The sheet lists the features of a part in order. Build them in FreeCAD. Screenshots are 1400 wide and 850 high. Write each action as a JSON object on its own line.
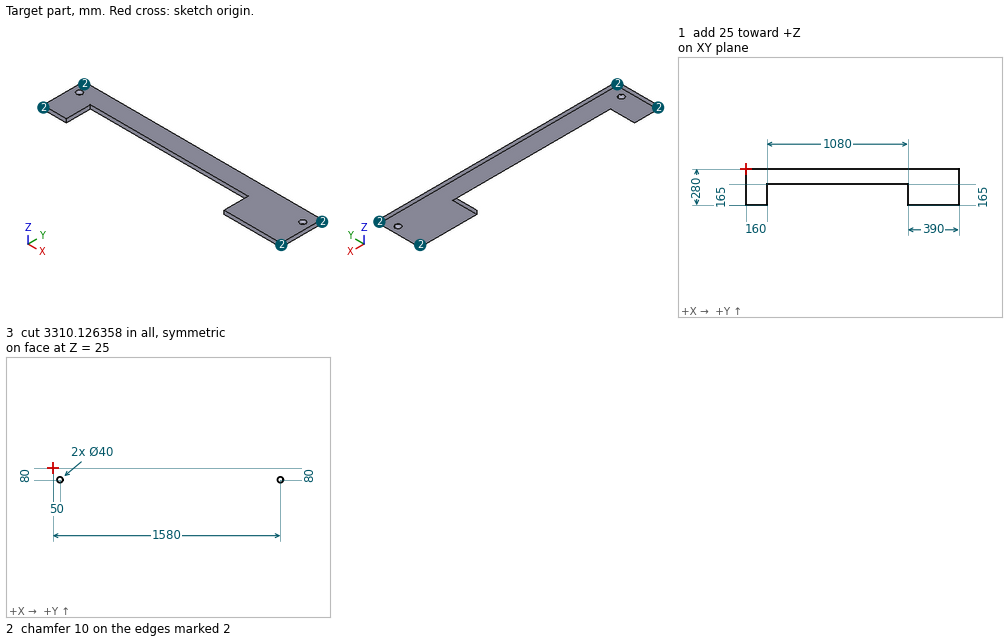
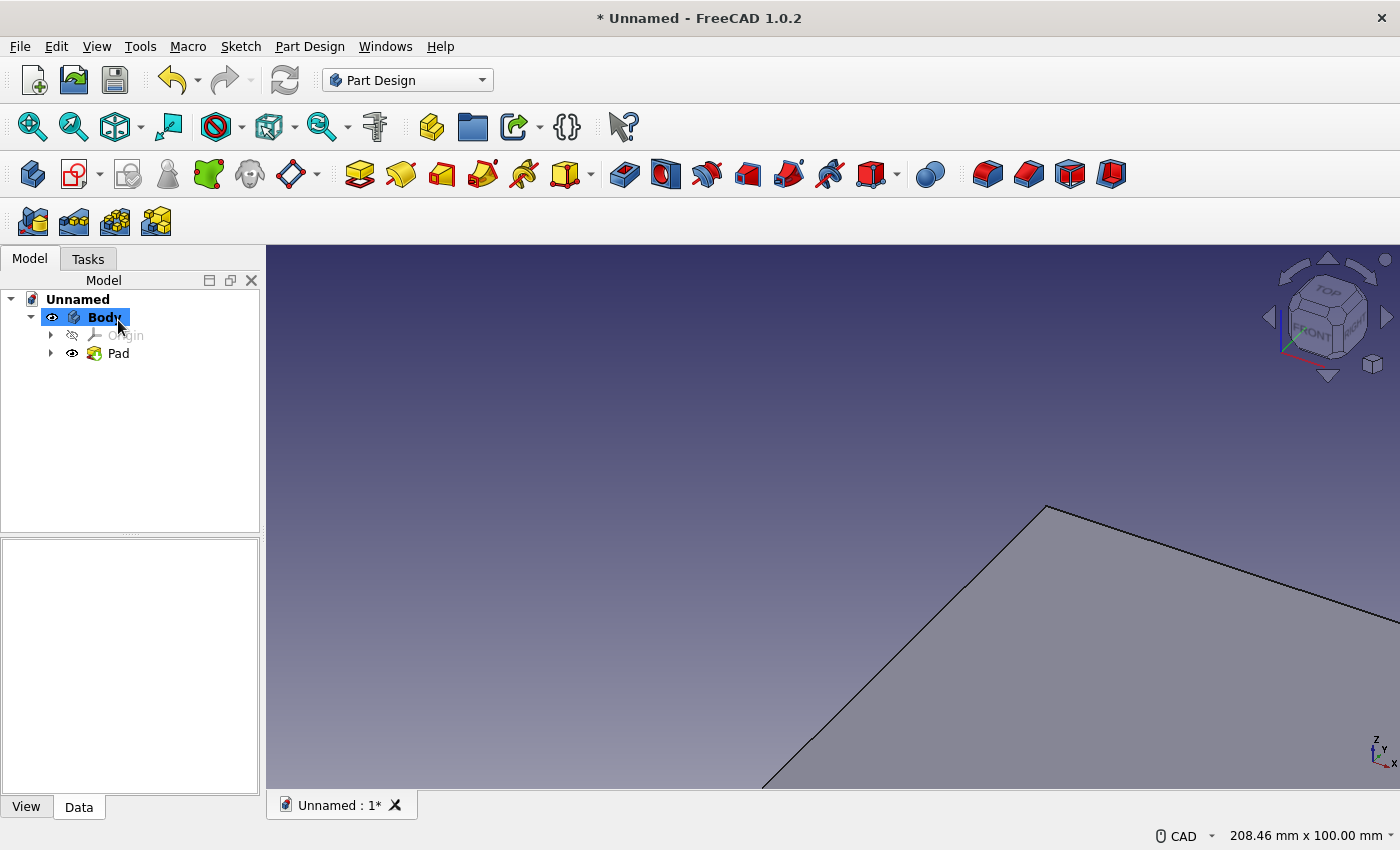
{"action": "key", "text": "v f"}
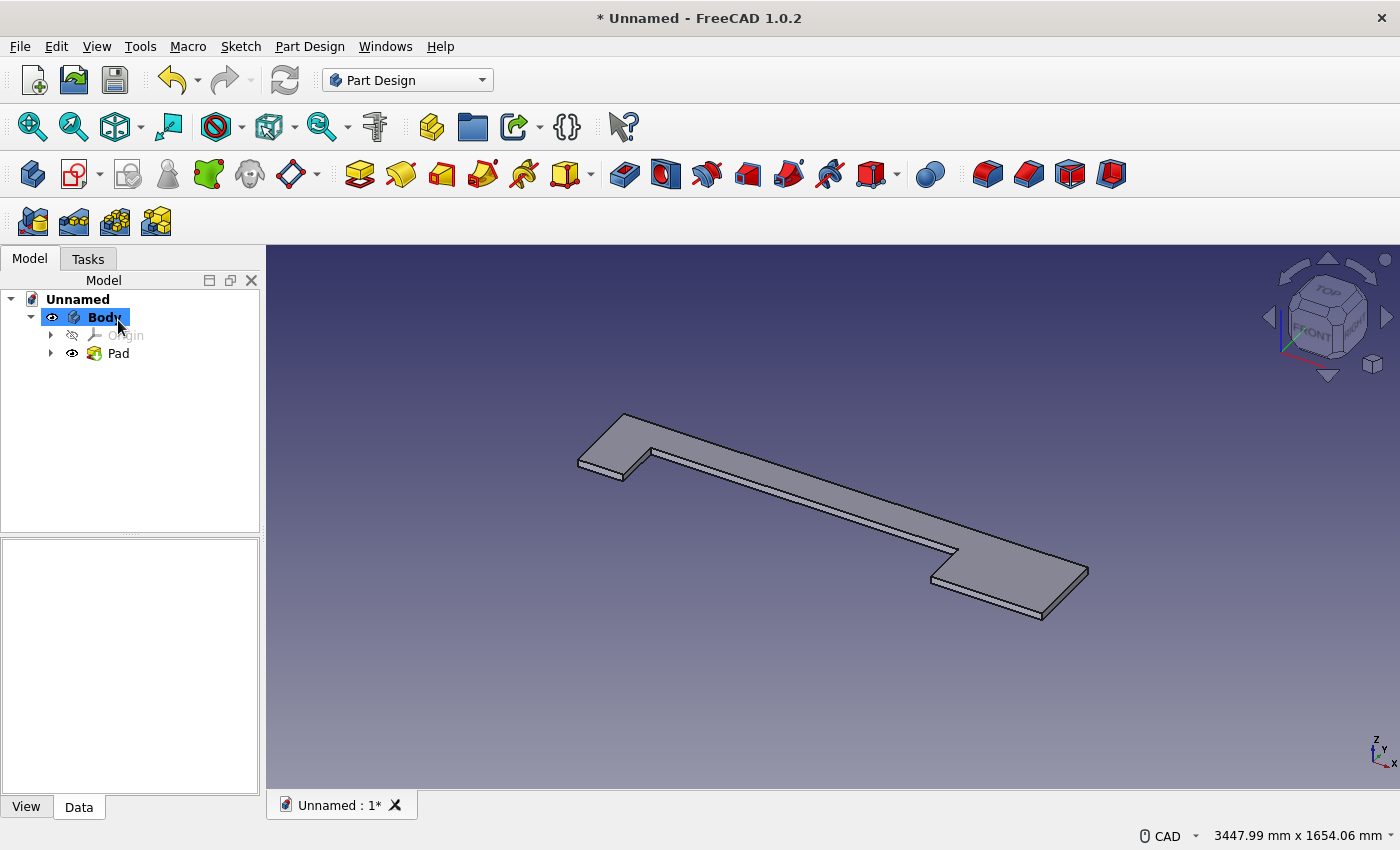
{"action": "scroll", "coordinate": [578, 462], "scroll_direction": "up", "scroll_amount": 8}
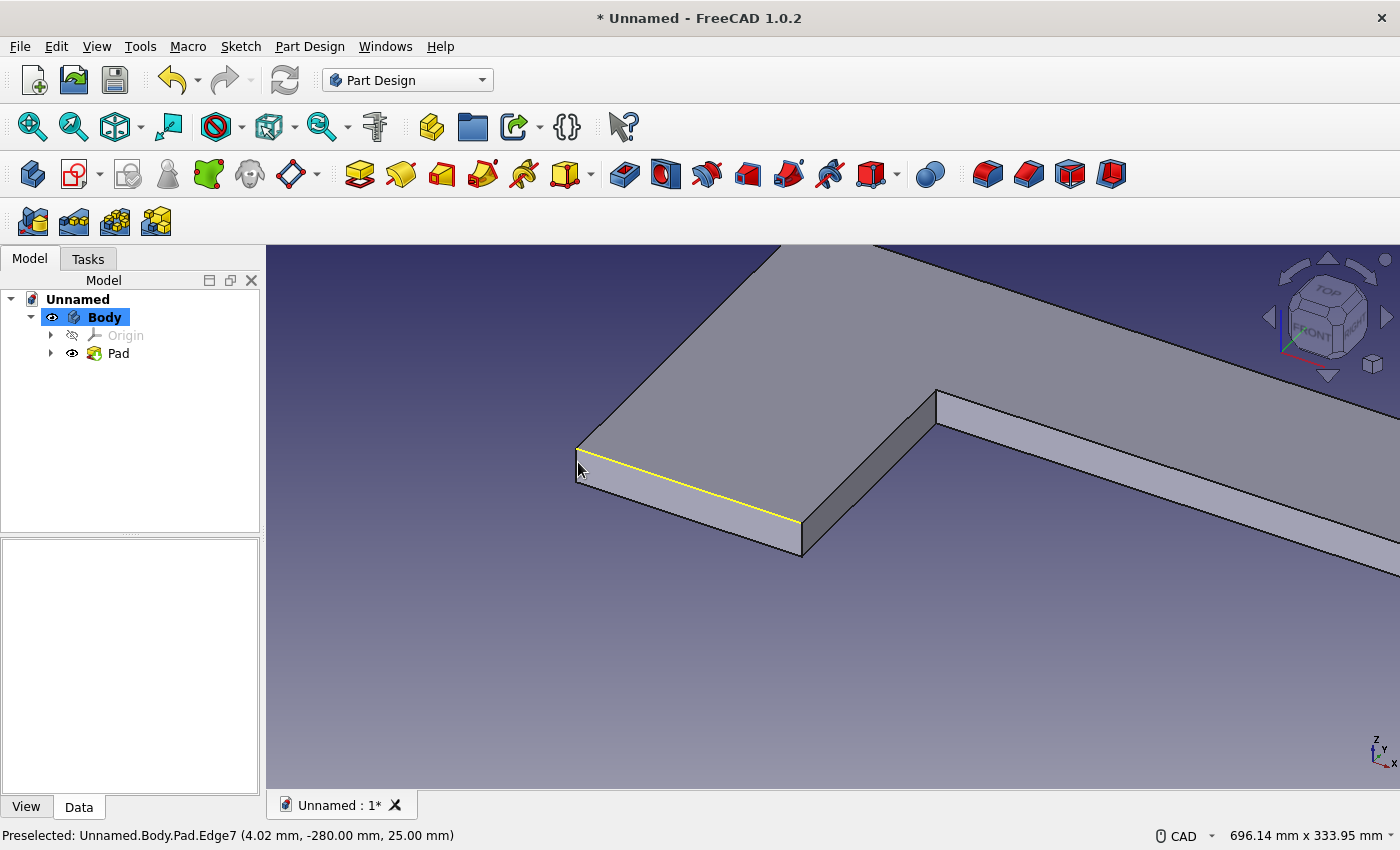
{"action": "key", "text": "v f"}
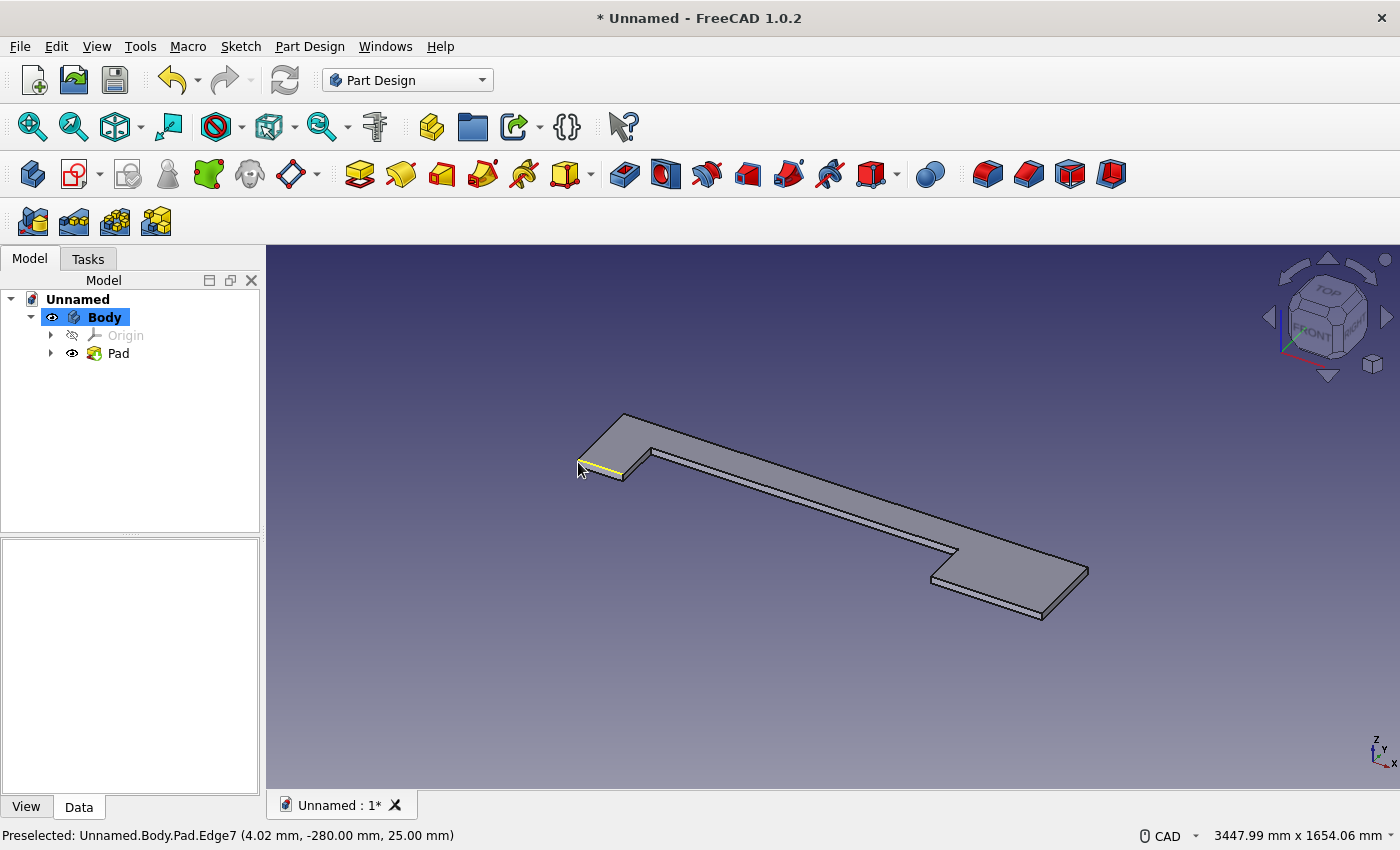
{"action": "key", "text": "0"}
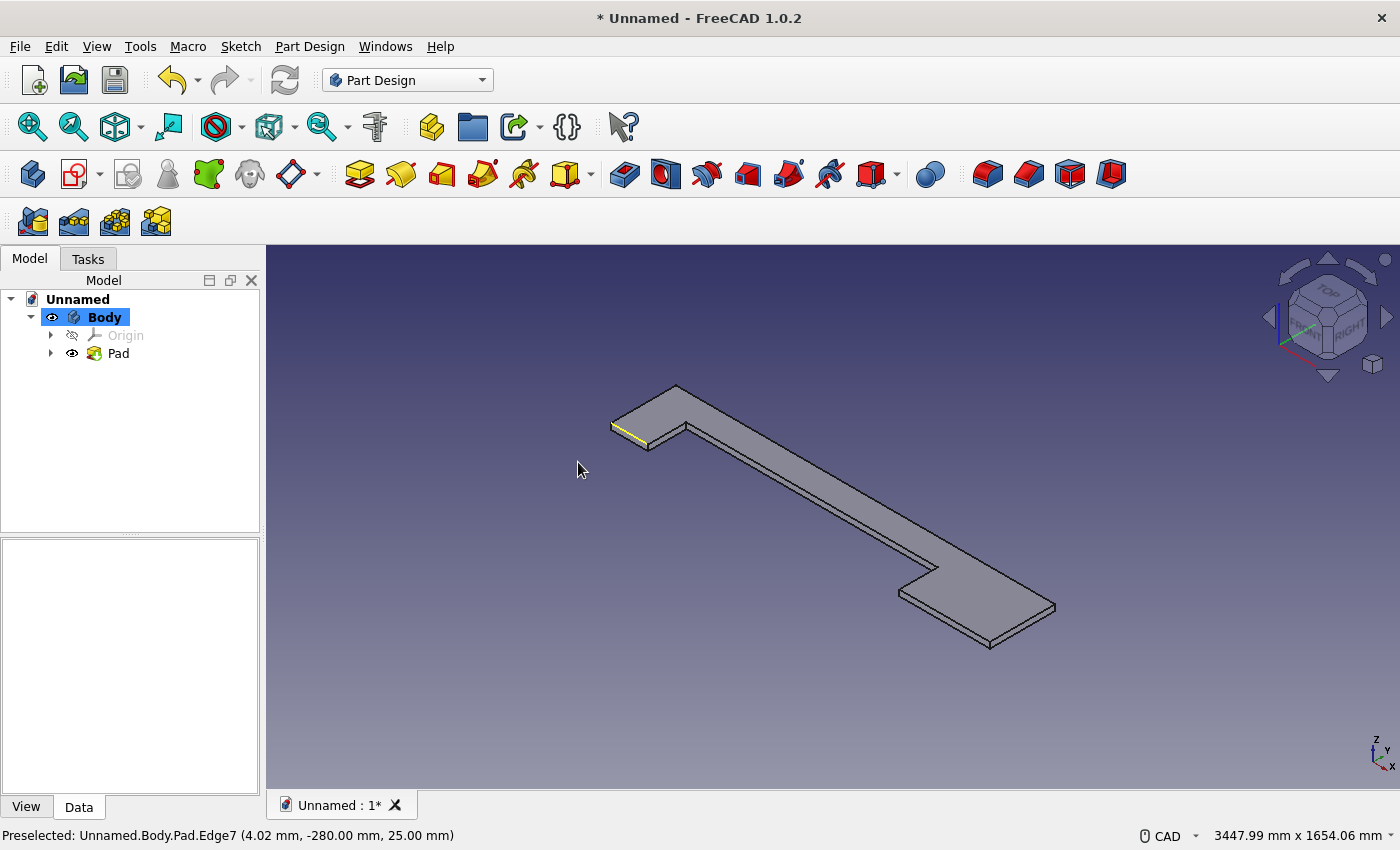
{"action": "scroll", "coordinate": [611, 425], "scroll_direction": "up", "scroll_amount": 8}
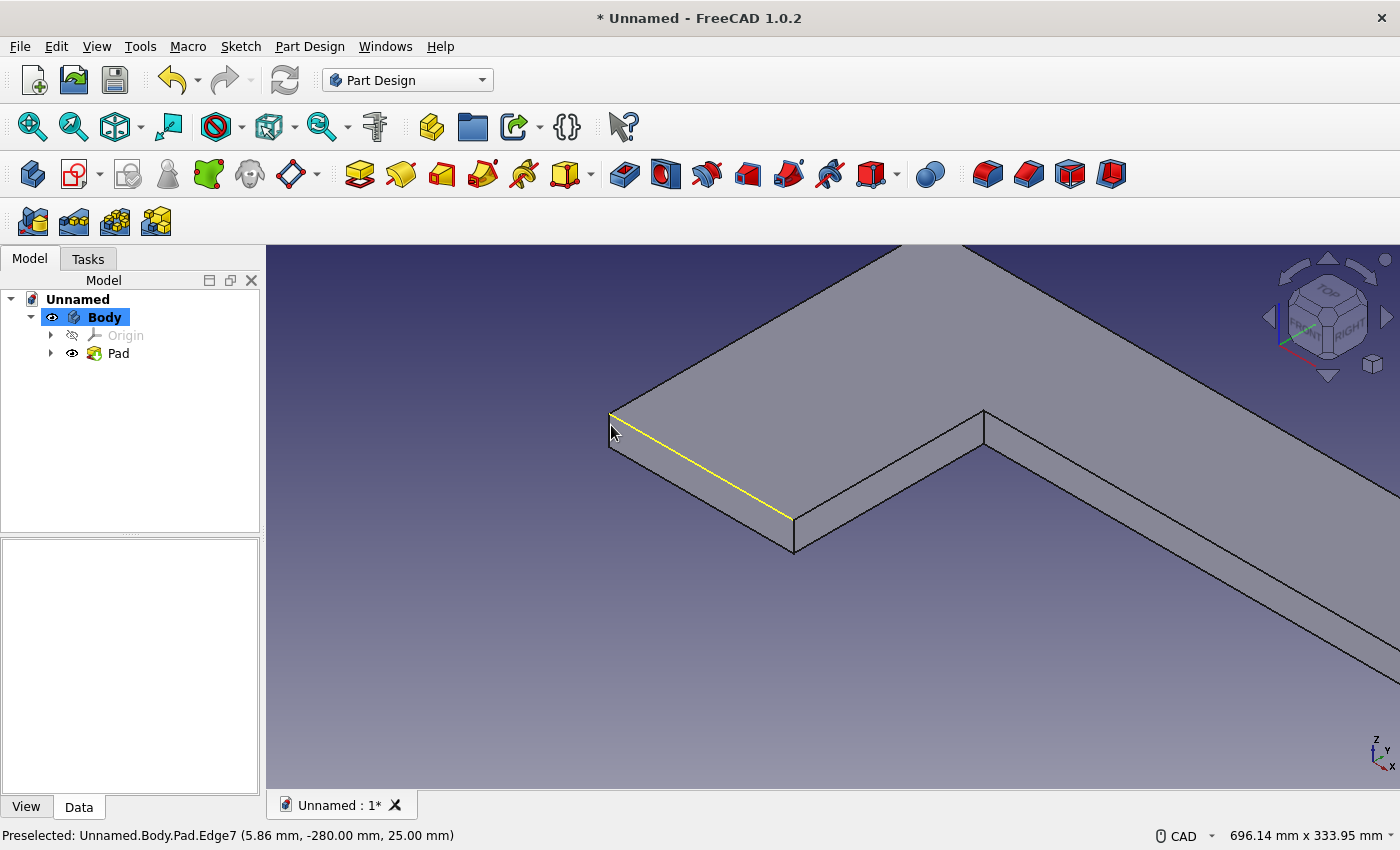
{"action": "key", "text": "v f"}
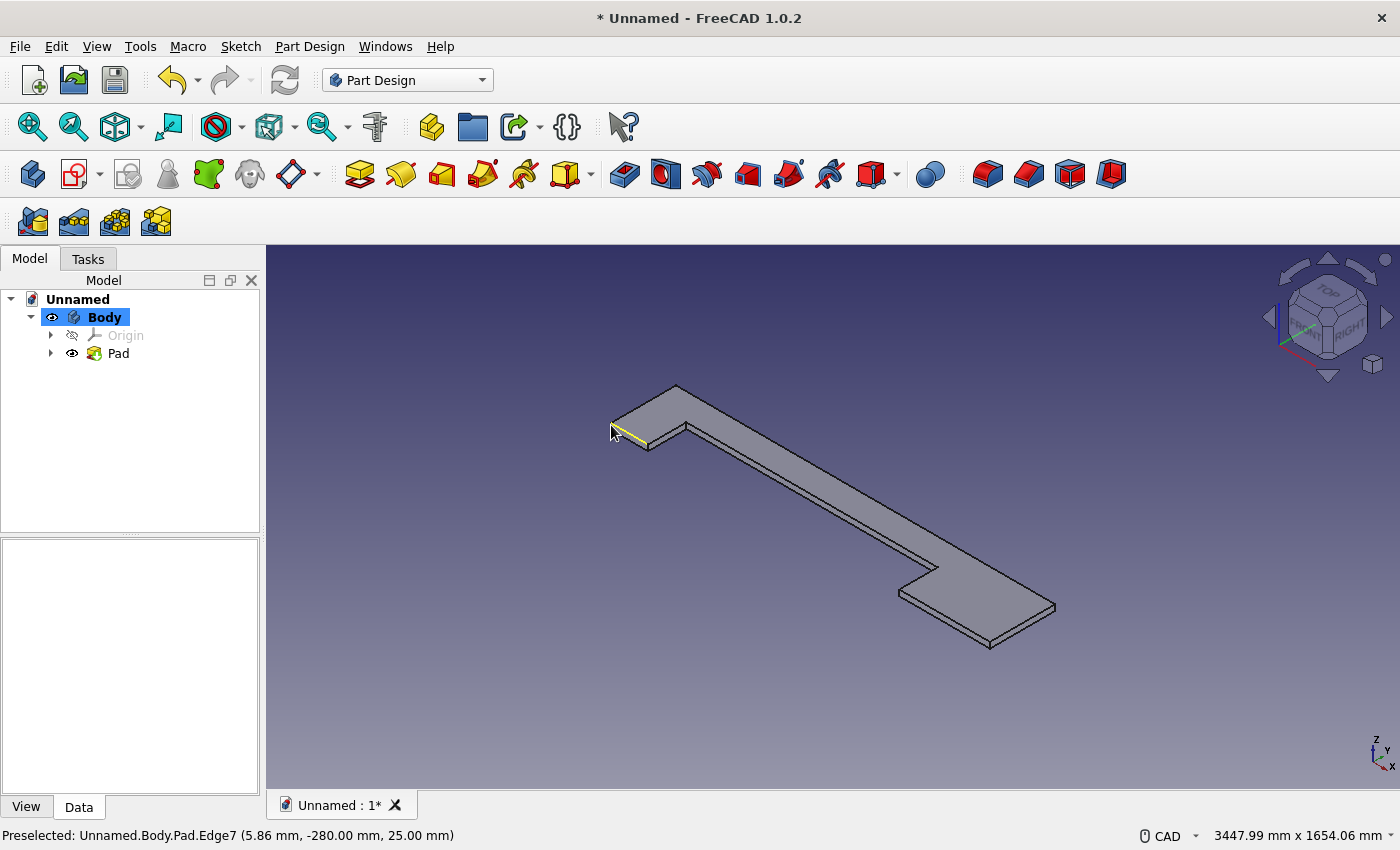
{"action": "key", "text": "2"}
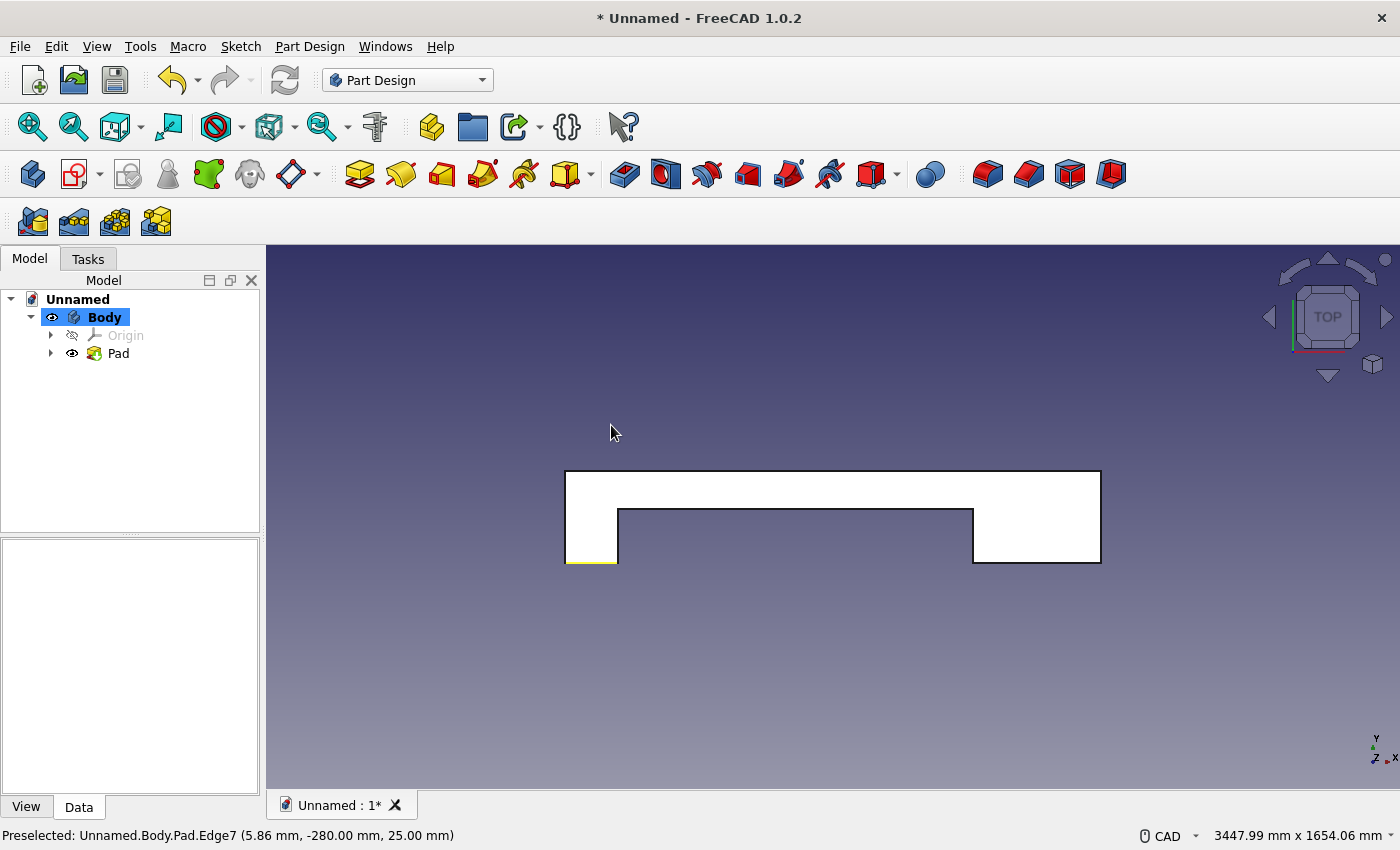
{"action": "scroll", "coordinate": [565, 562], "scroll_direction": "up", "scroll_amount": 8}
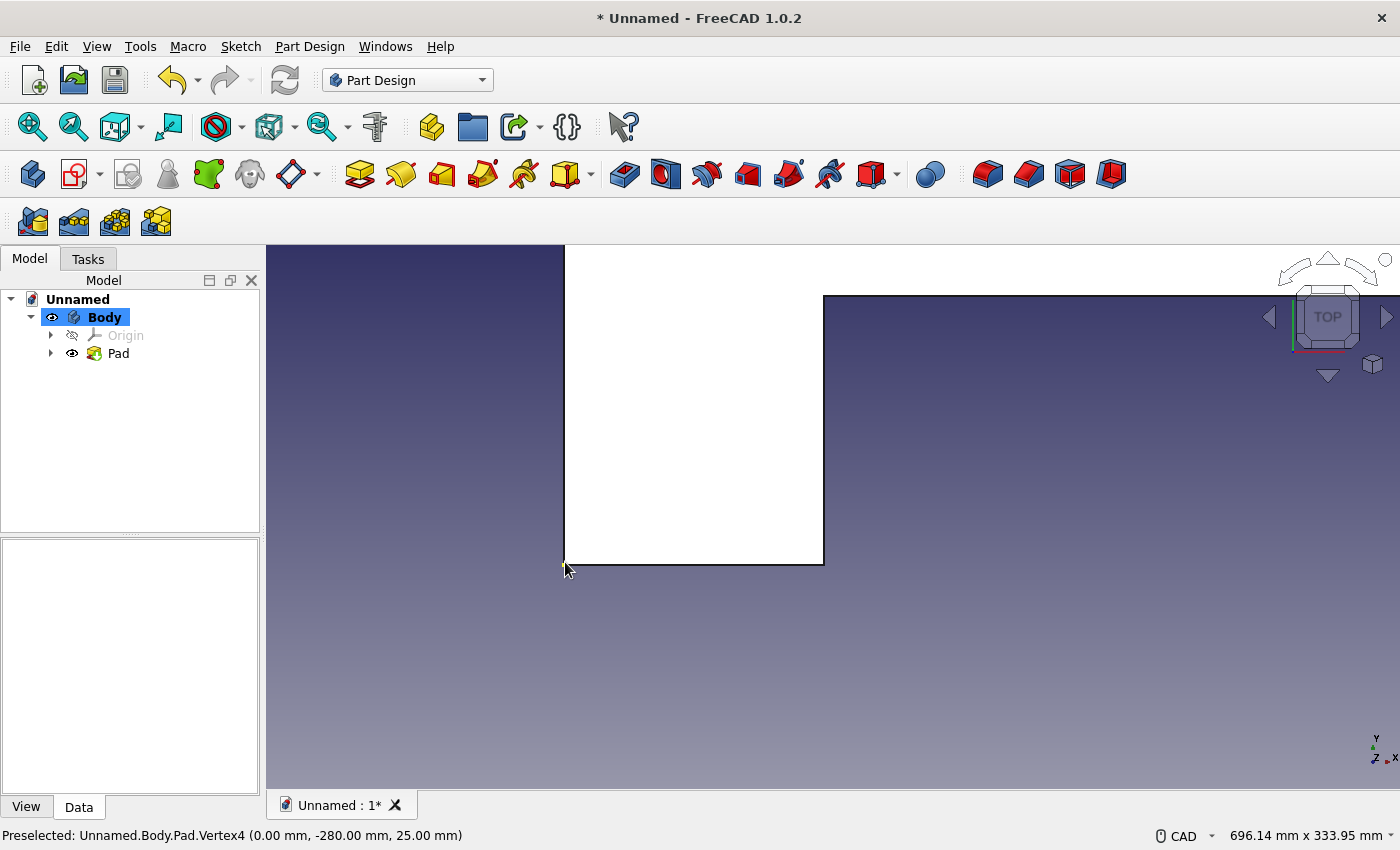
{"action": "left_click", "coordinate": [33, 128]}